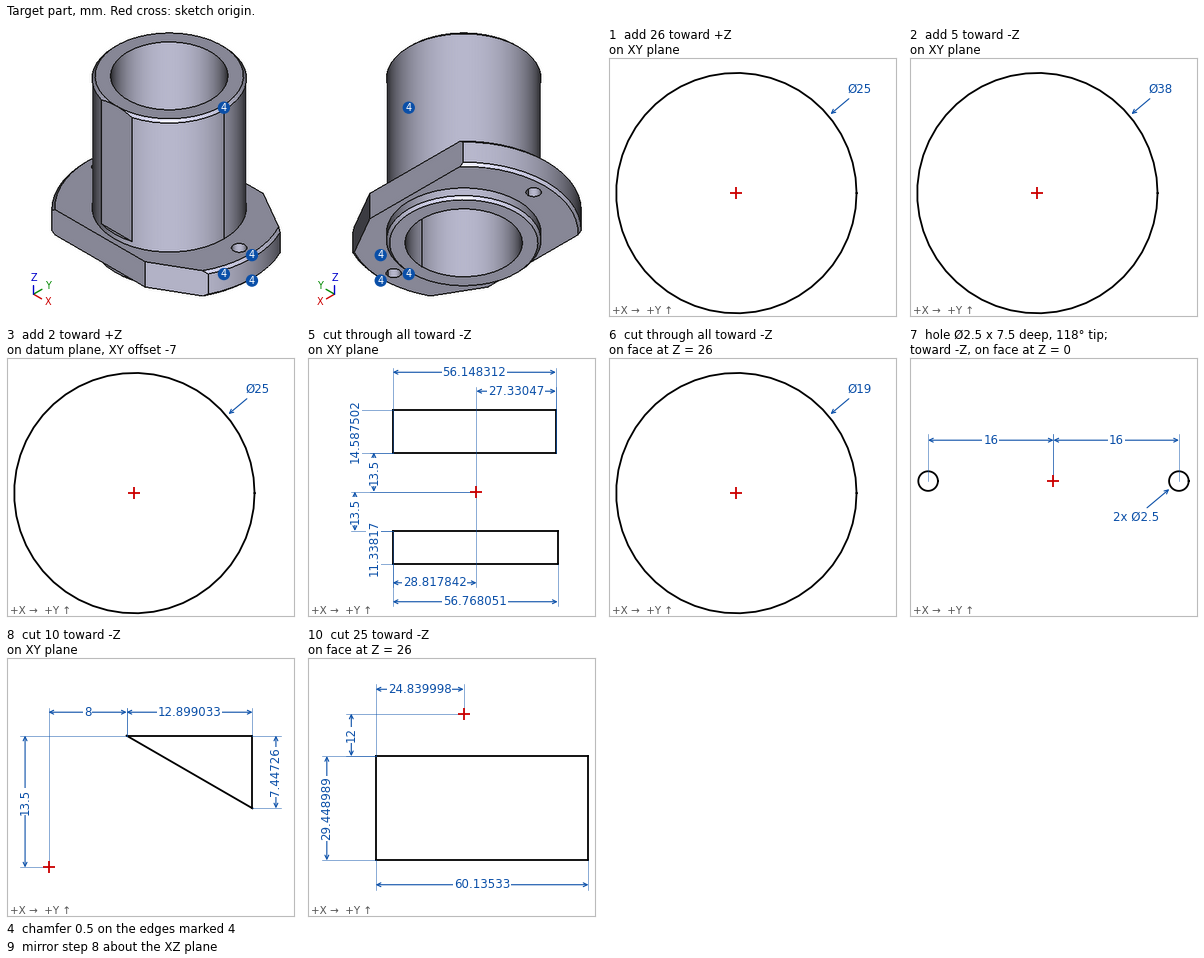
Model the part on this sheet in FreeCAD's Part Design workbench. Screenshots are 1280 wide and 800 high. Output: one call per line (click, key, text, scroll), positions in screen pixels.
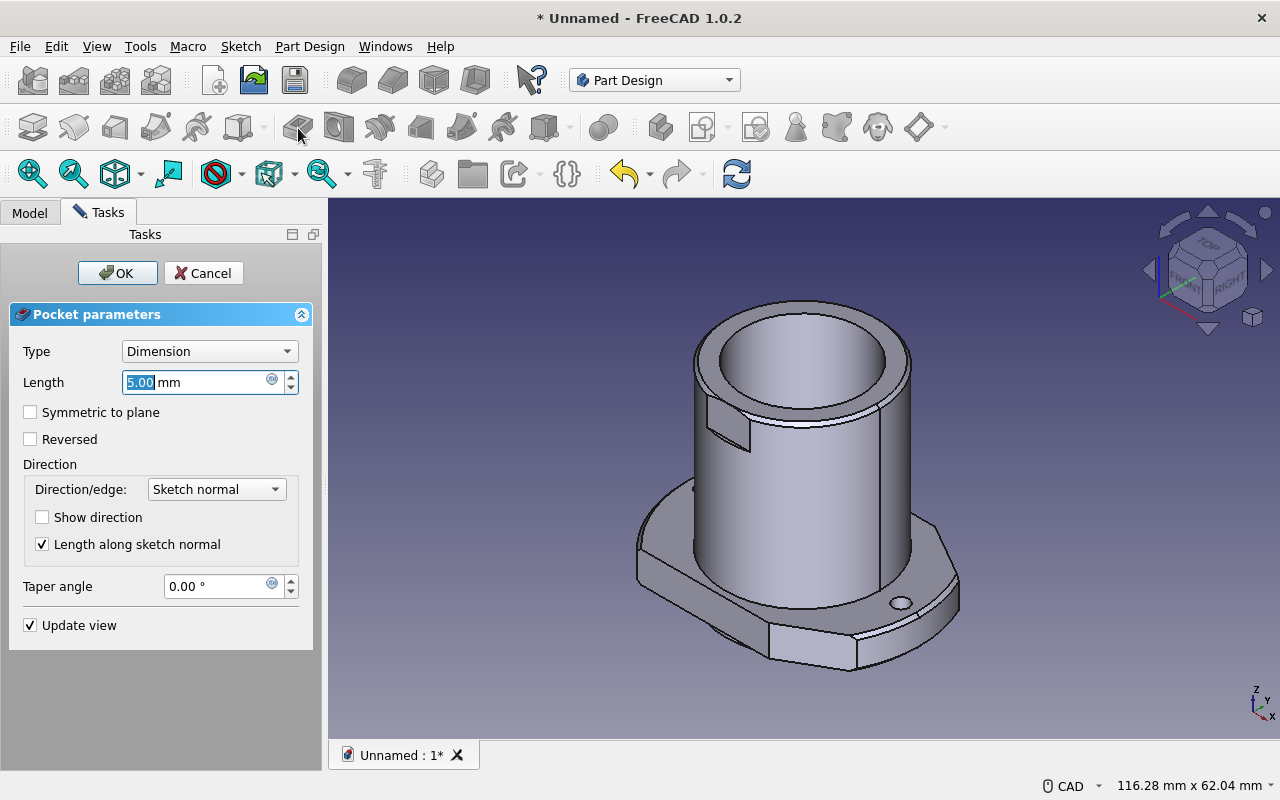
text(25)
key(Tab)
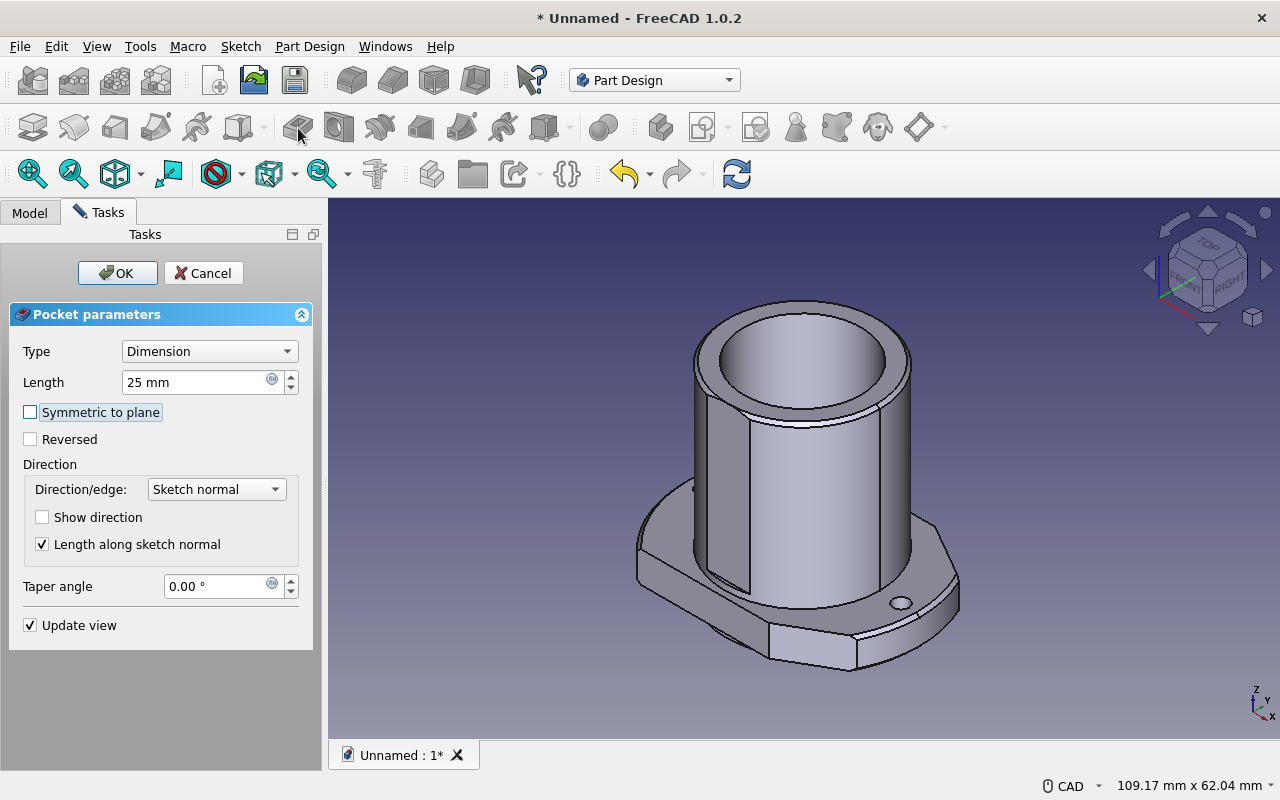
click(118, 273)